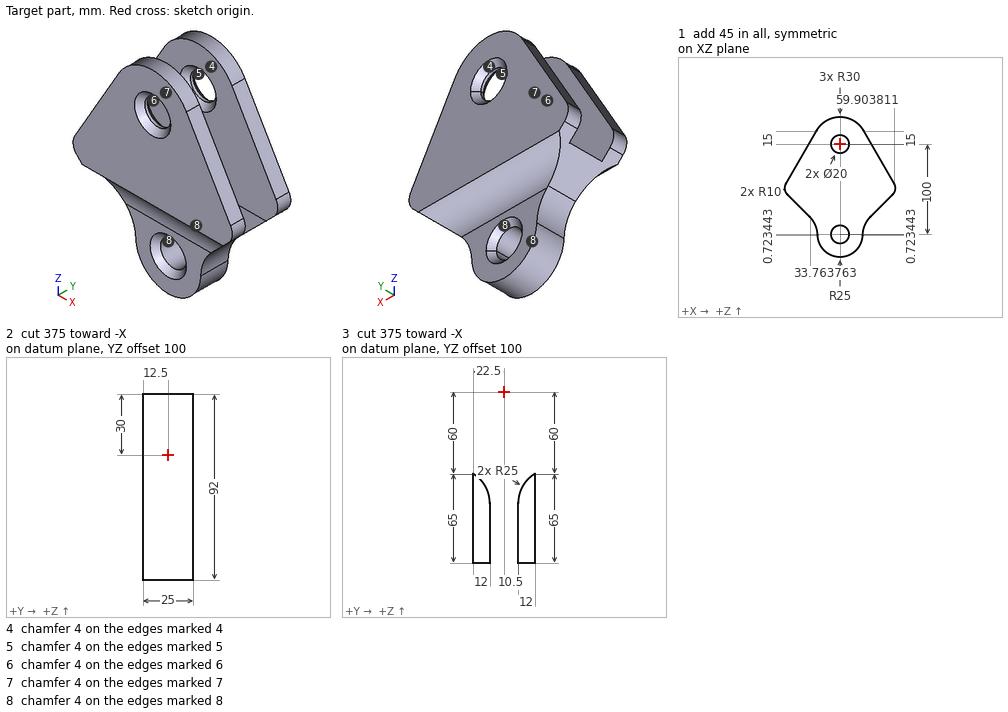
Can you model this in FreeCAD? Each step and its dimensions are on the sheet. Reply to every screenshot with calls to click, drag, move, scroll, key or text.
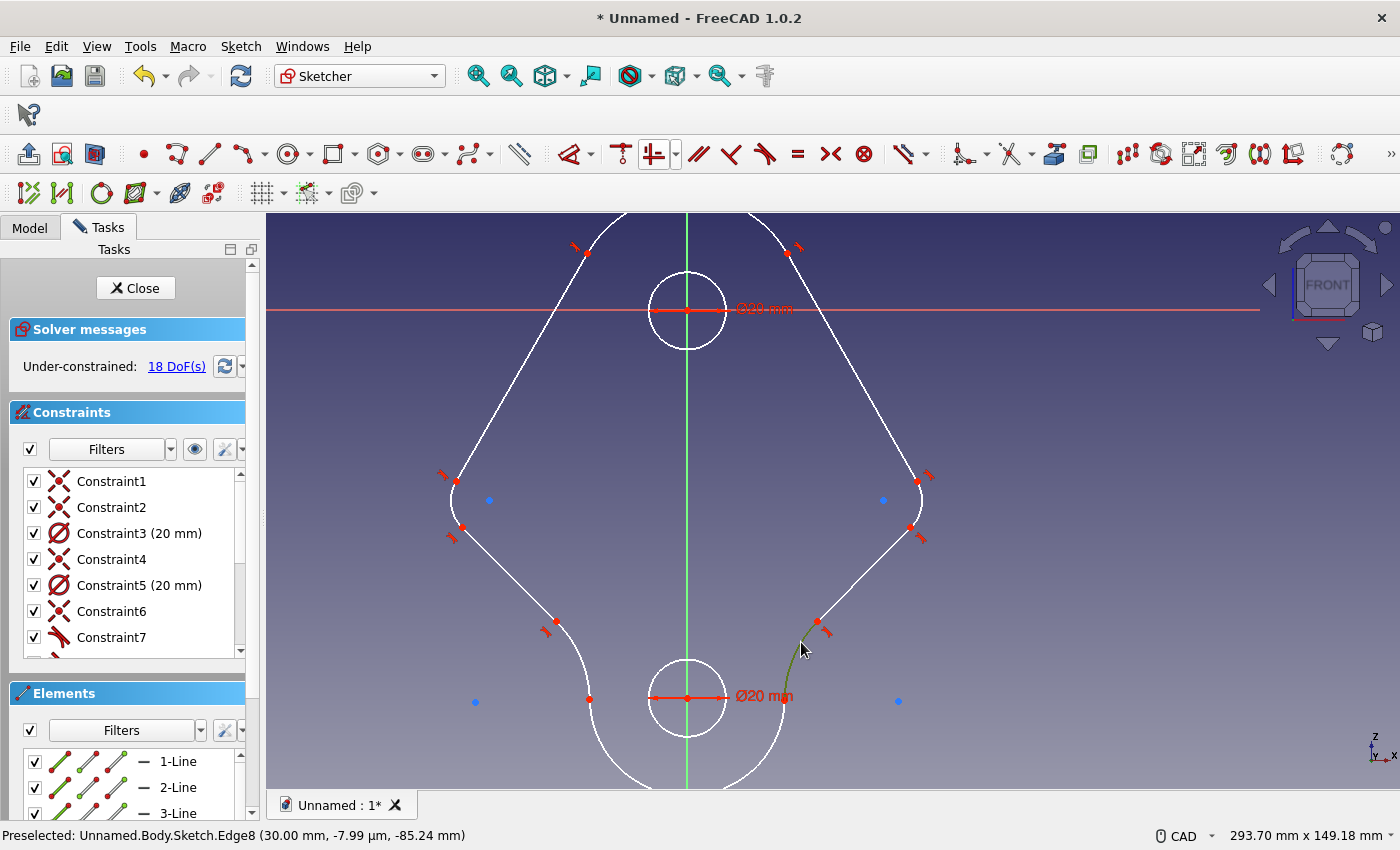
click(609, 756)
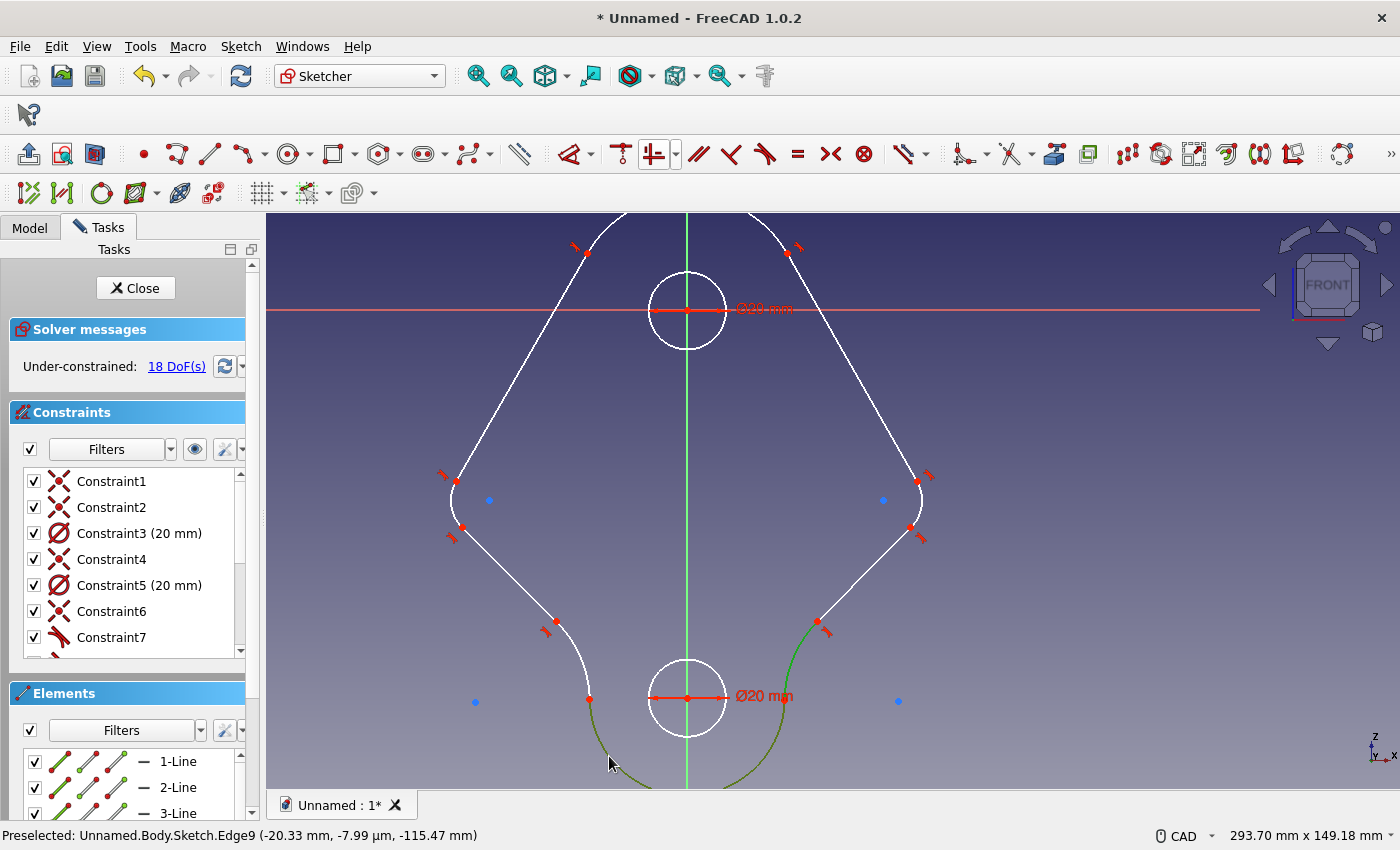
click(765, 154)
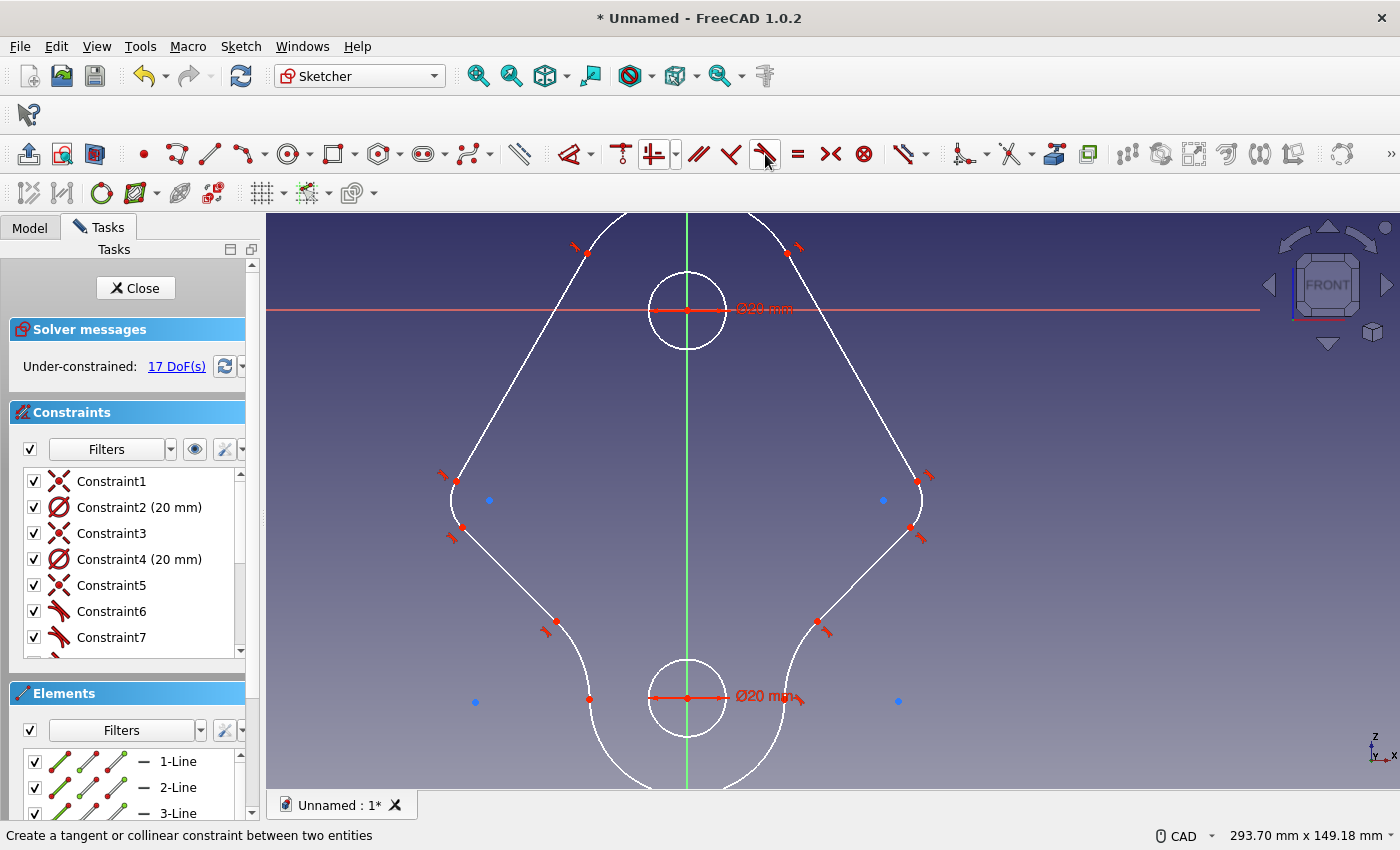
click(609, 756)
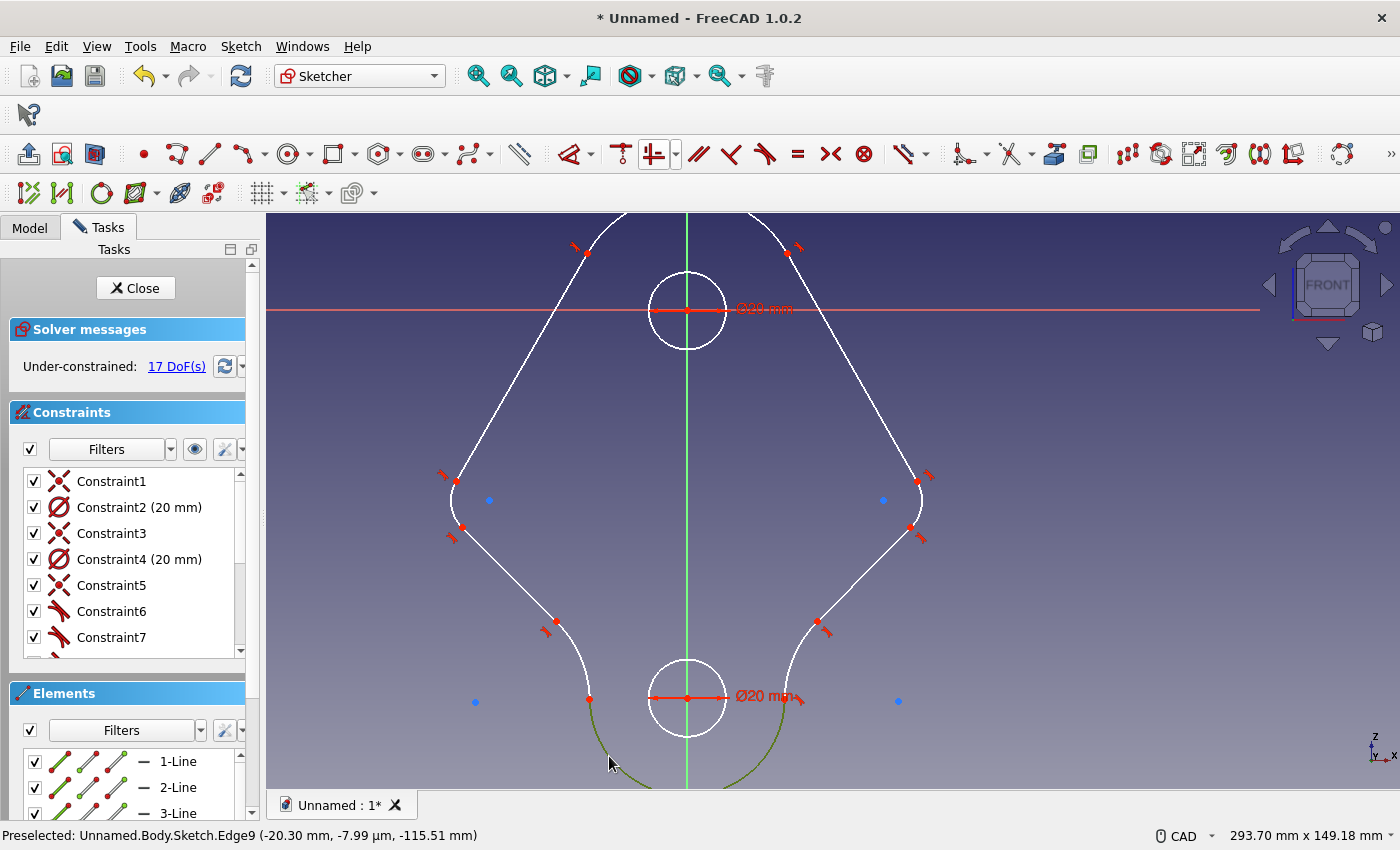
click(586, 674)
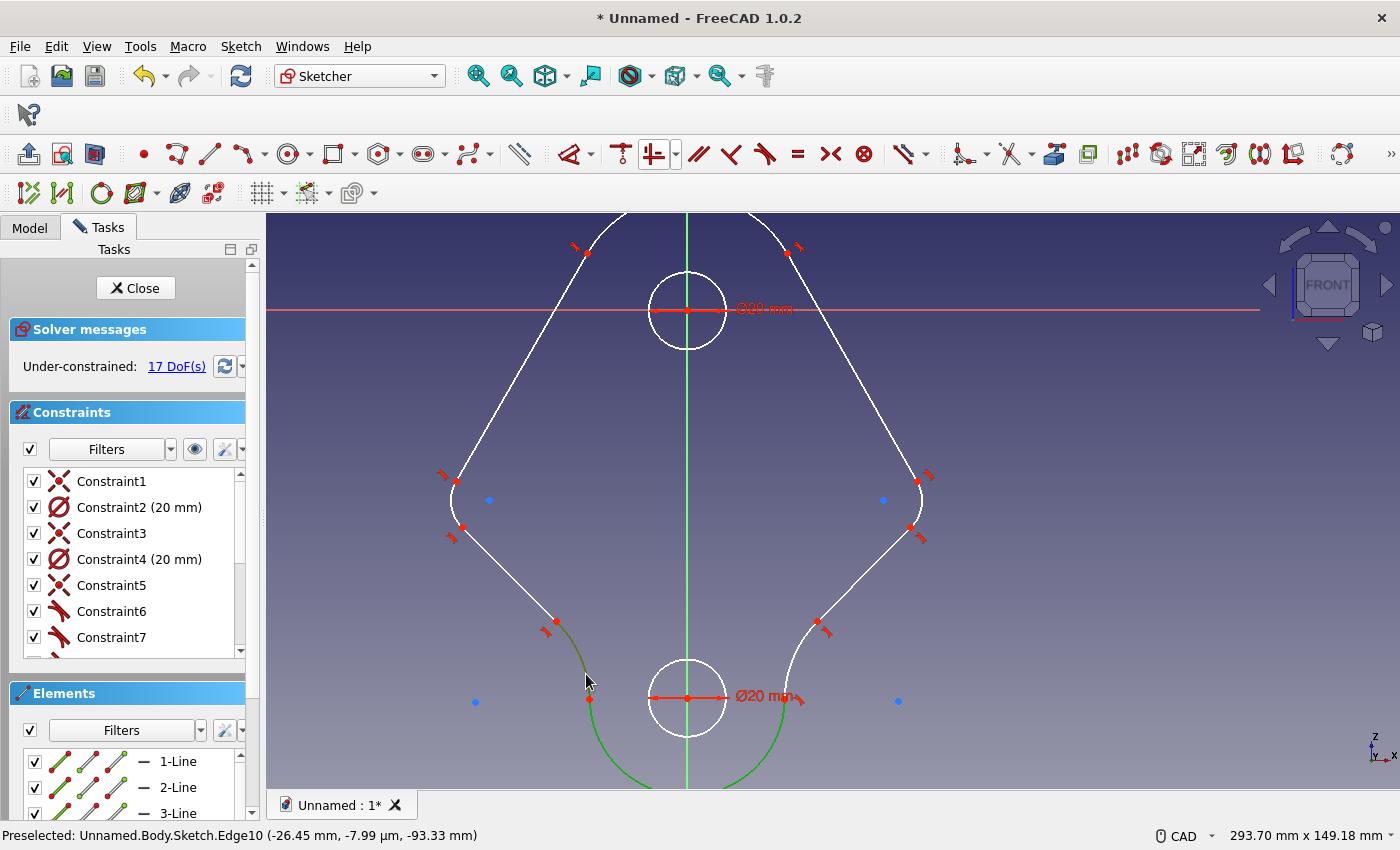
click(765, 154)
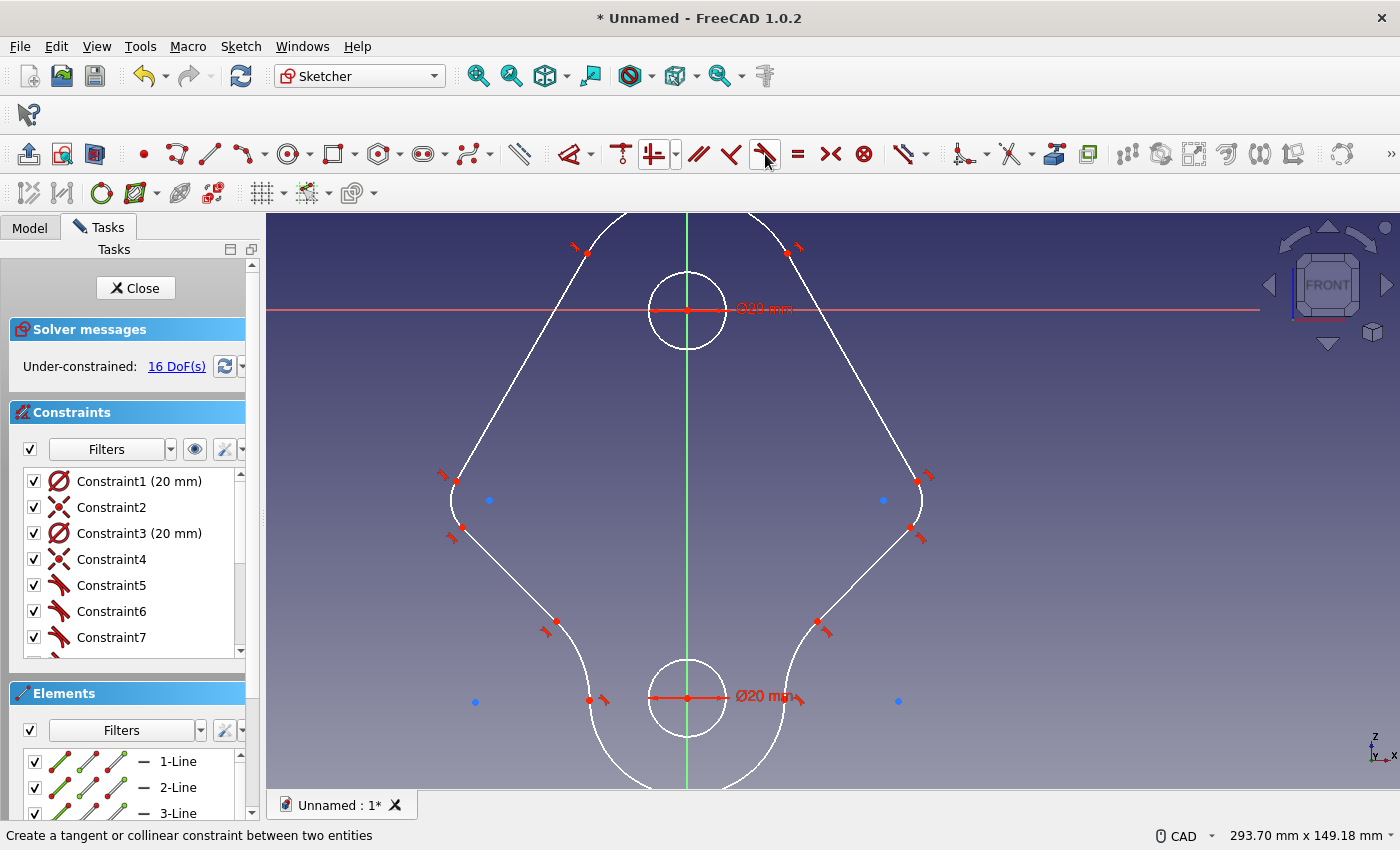
drag(677, 300, 697, 321)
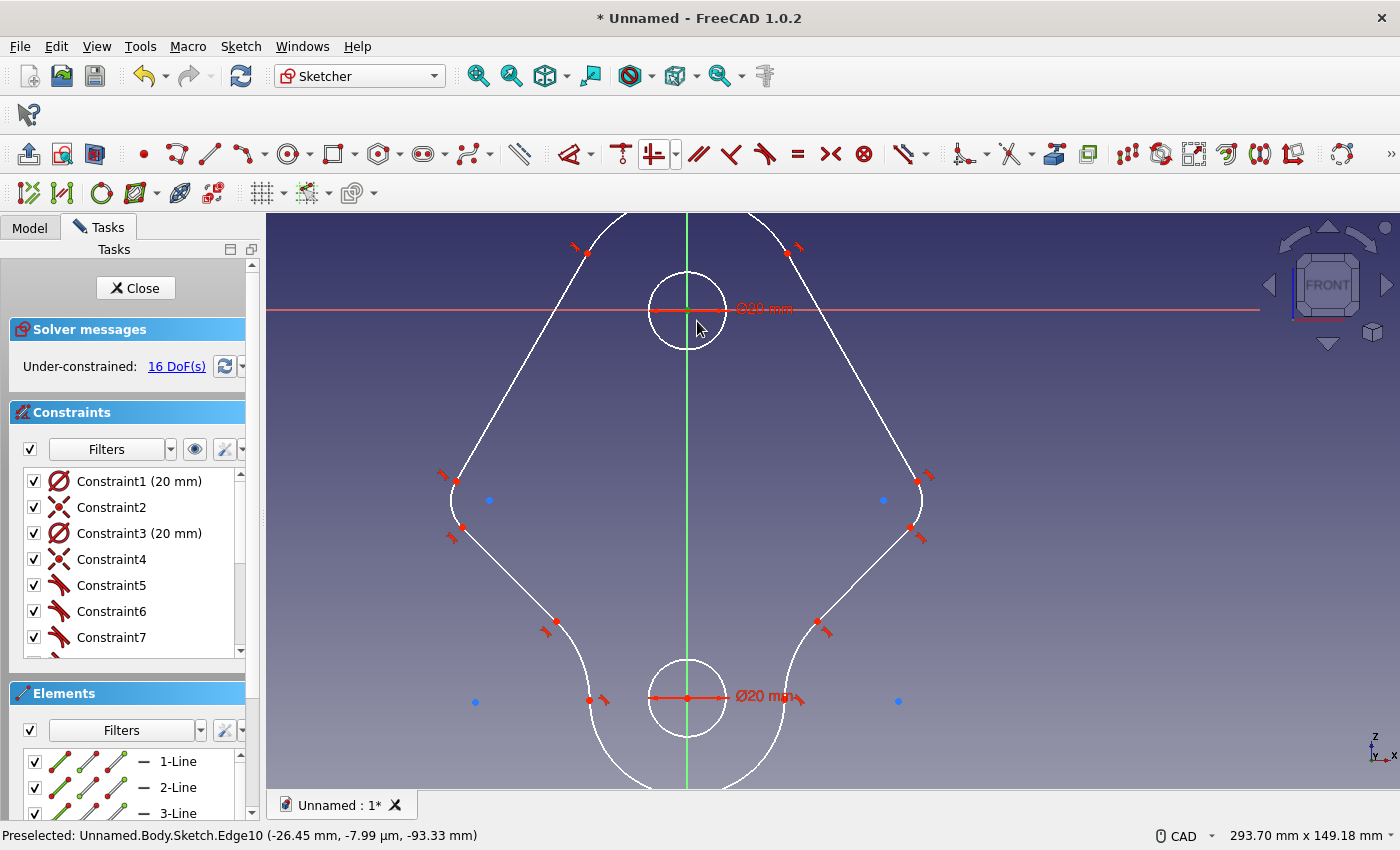
key(c)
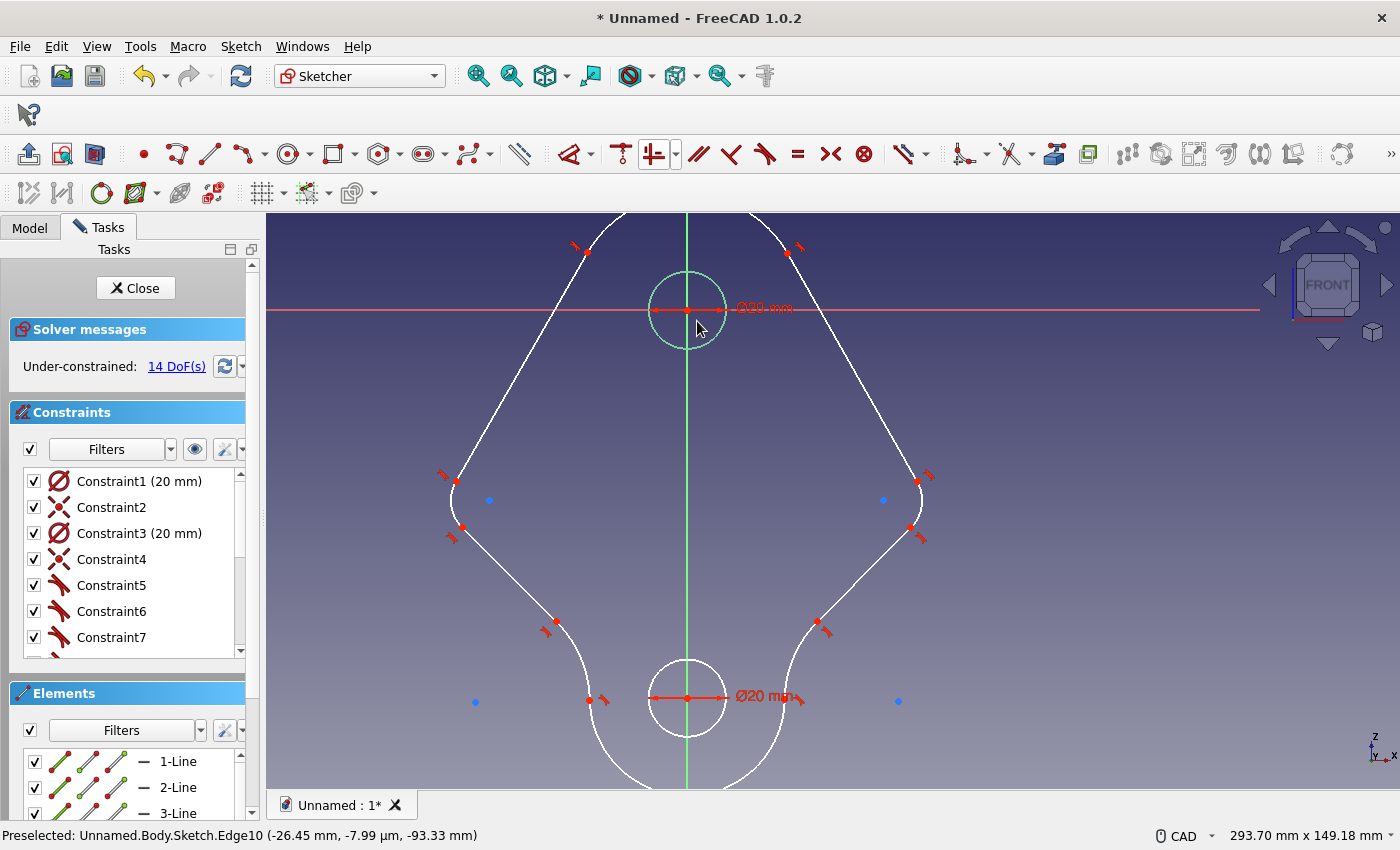
click(451, 496)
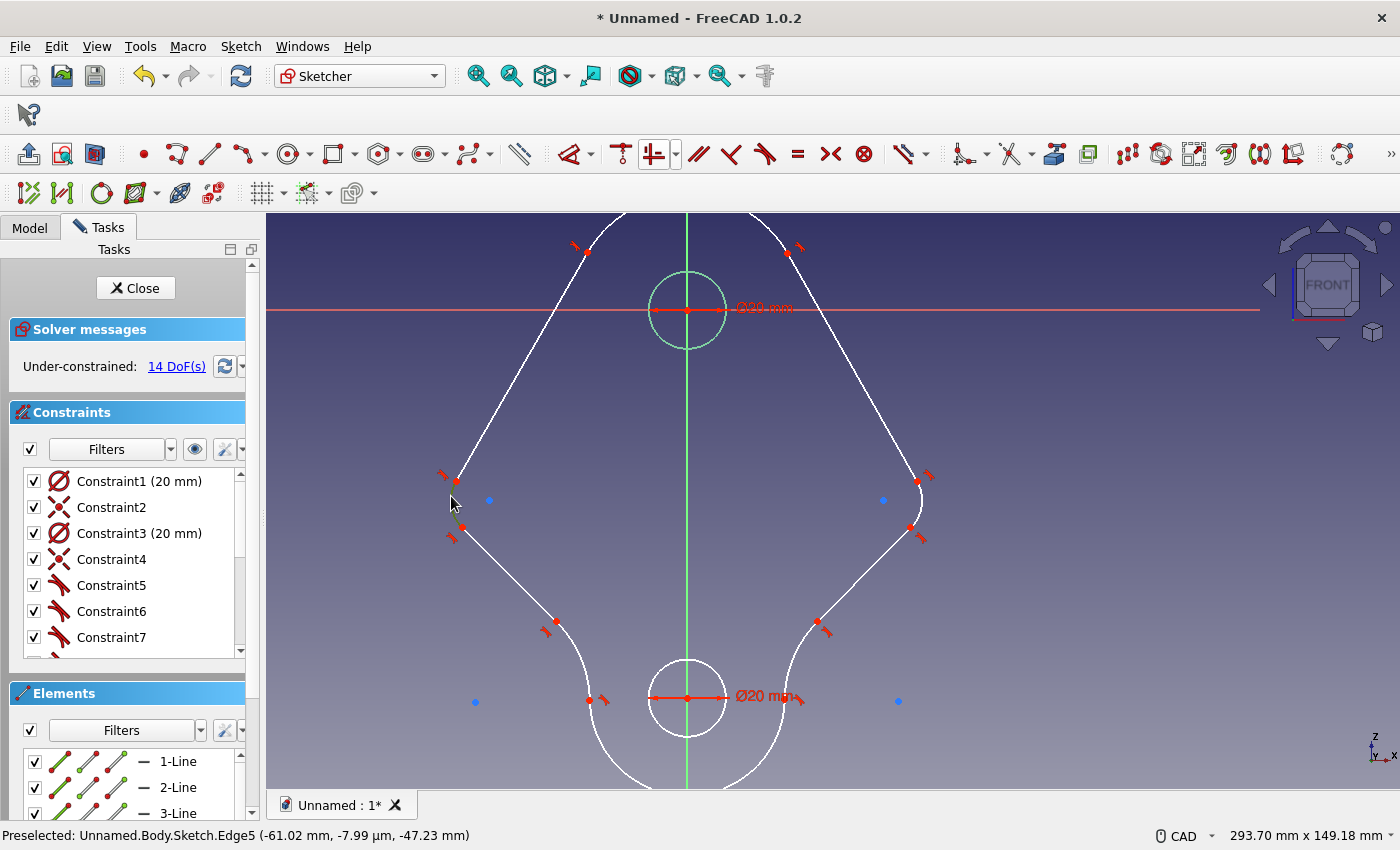
click(919, 515)